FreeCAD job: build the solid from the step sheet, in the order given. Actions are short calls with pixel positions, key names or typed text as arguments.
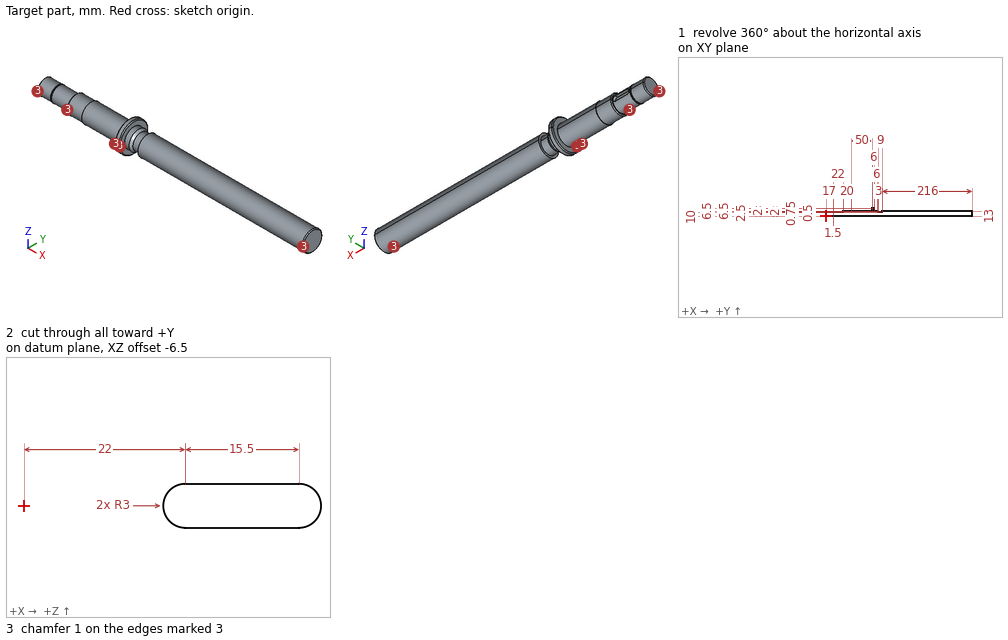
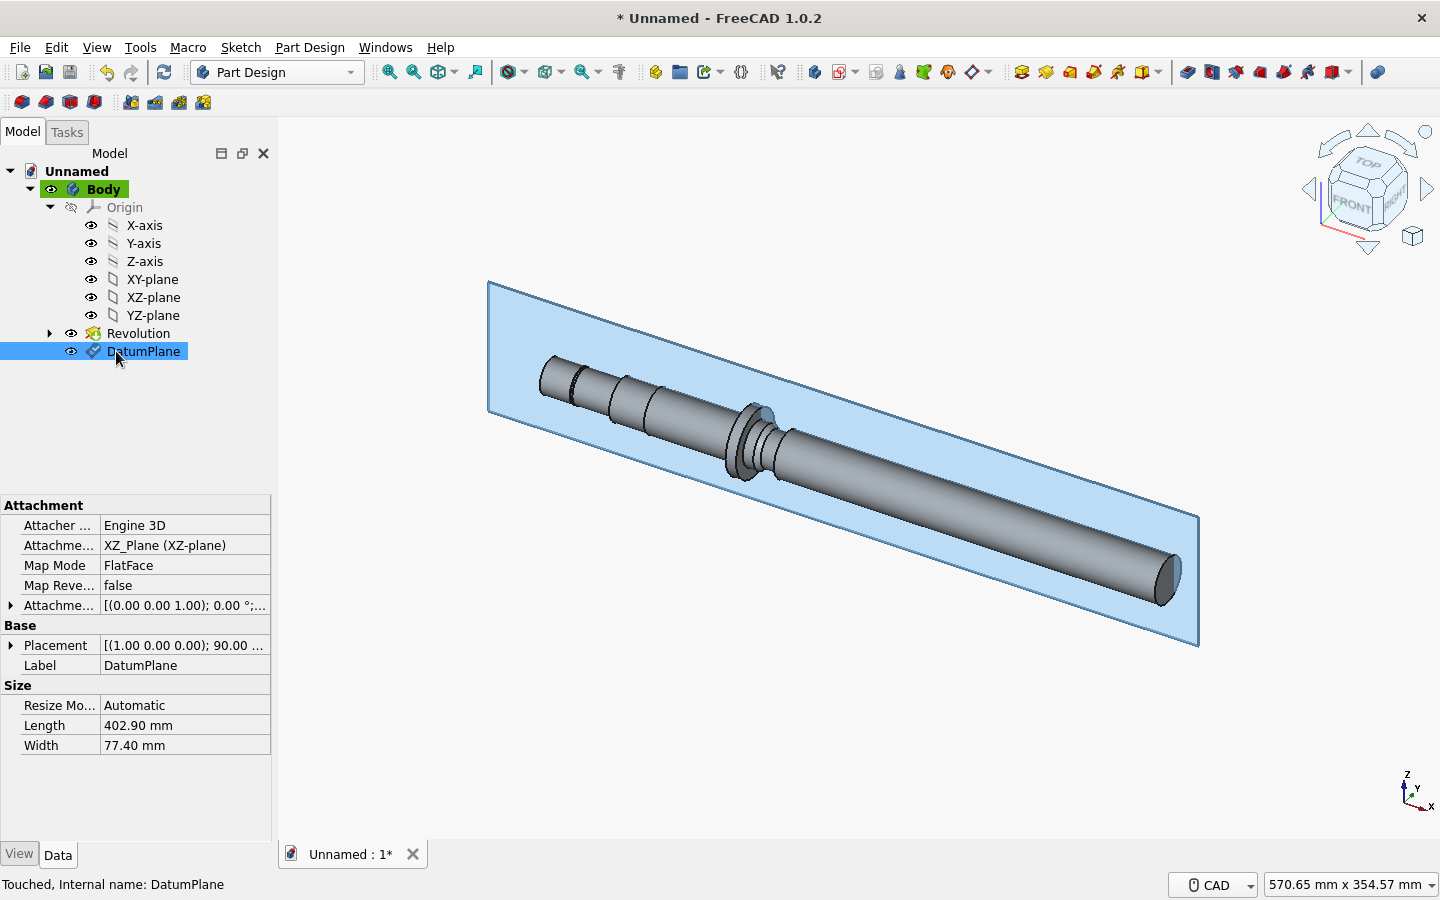
click(840, 72)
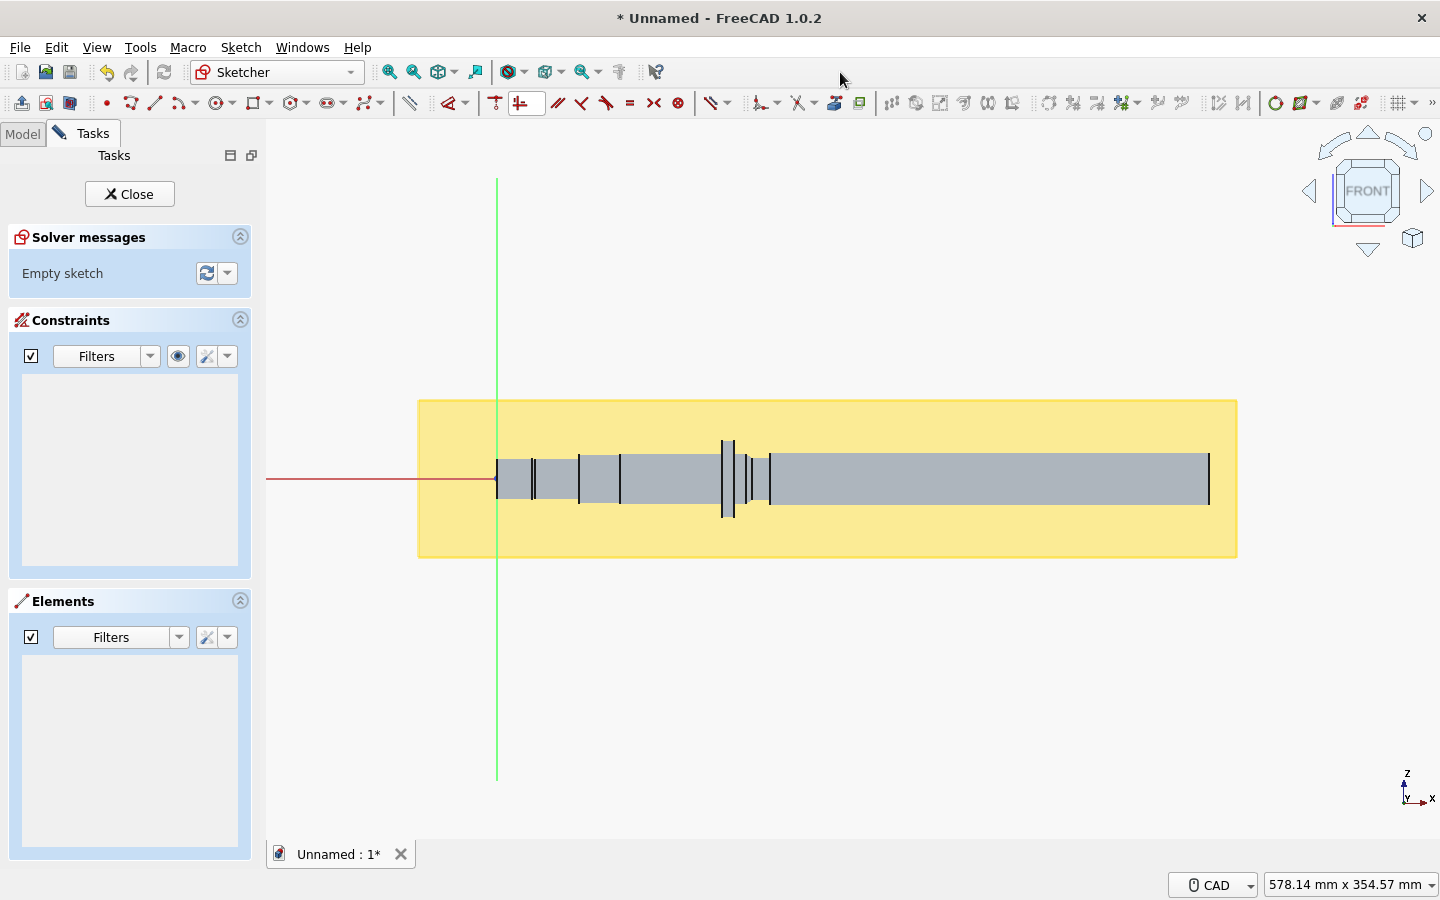
click(70, 104)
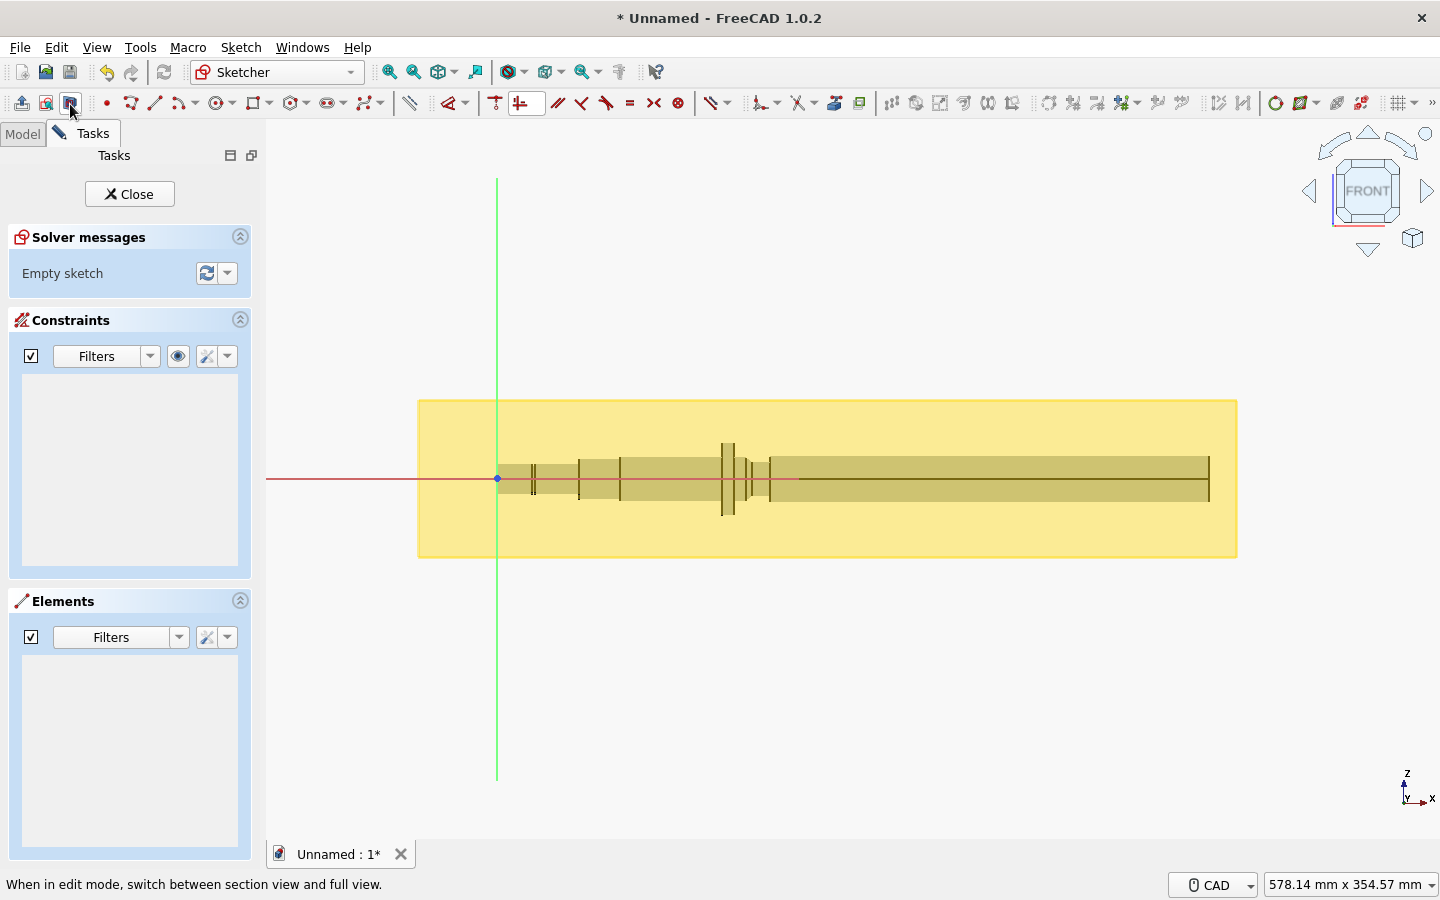
scroll(508, 479, up, 11)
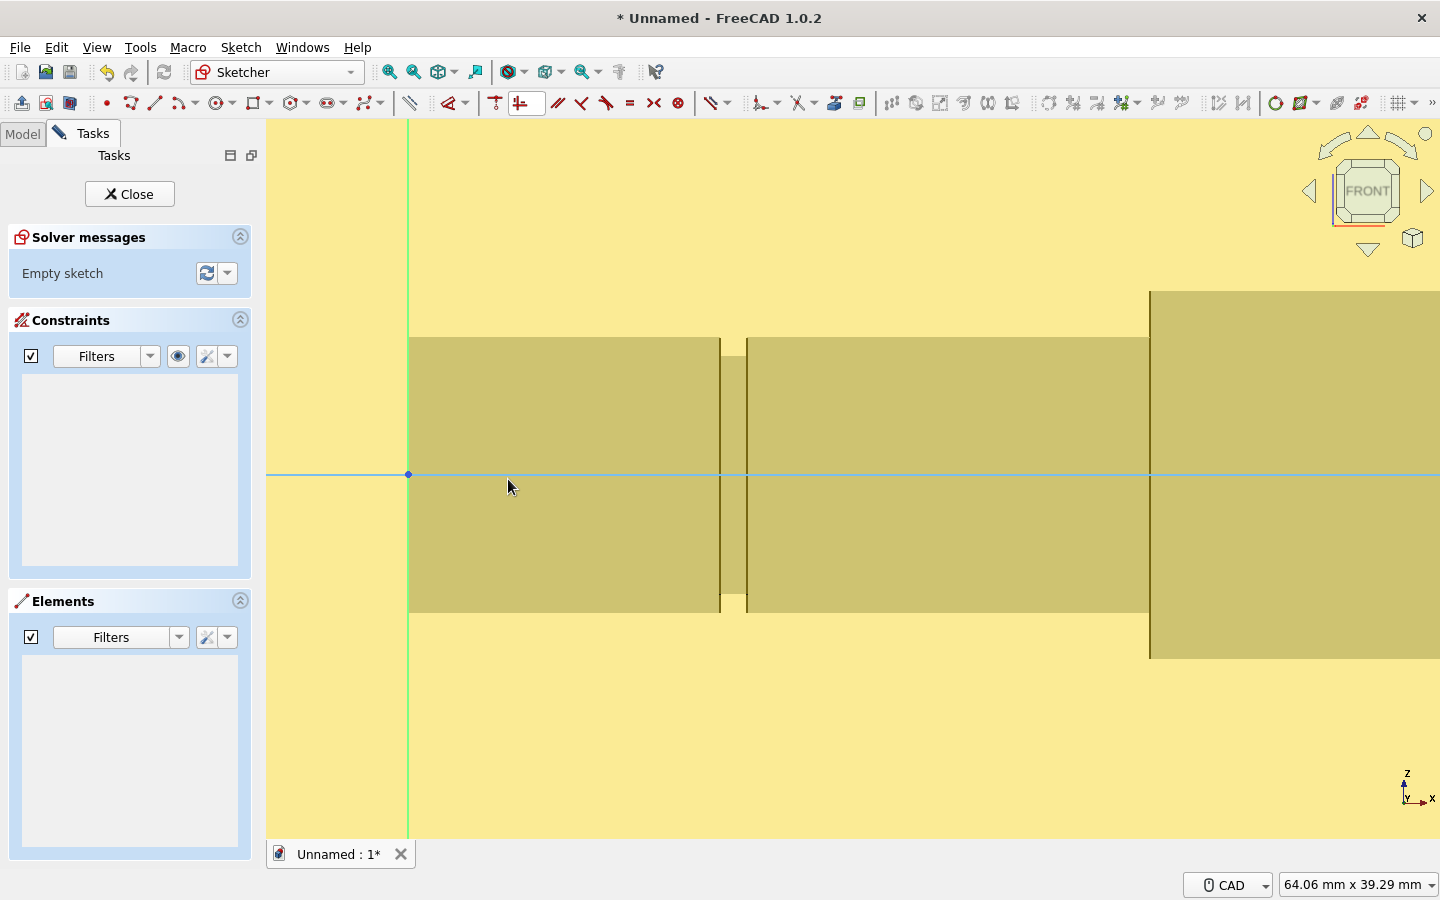
click(328, 104)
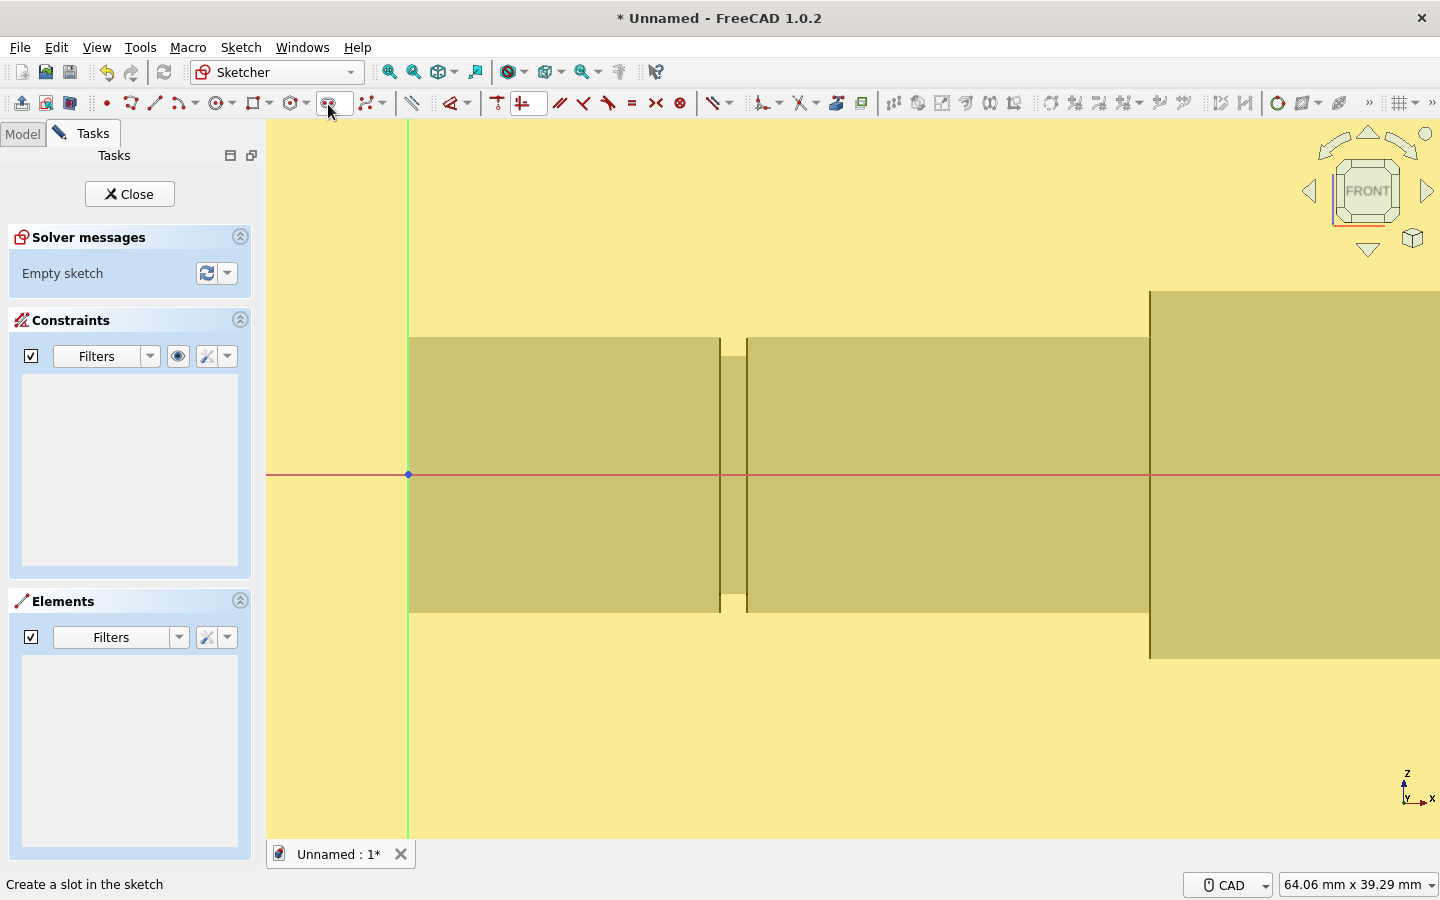
click(811, 475)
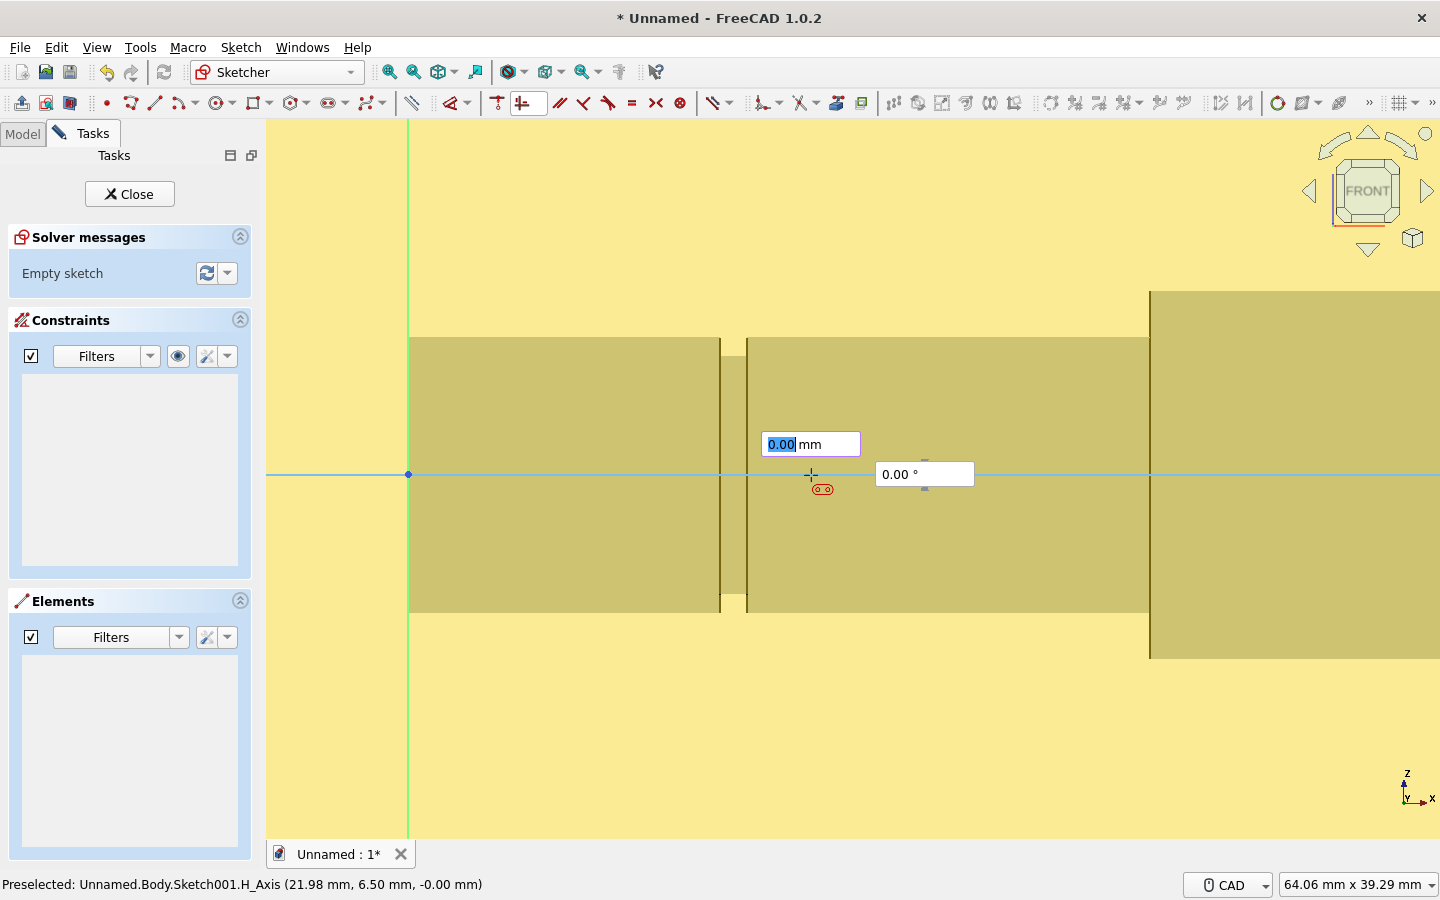
click(1095, 466)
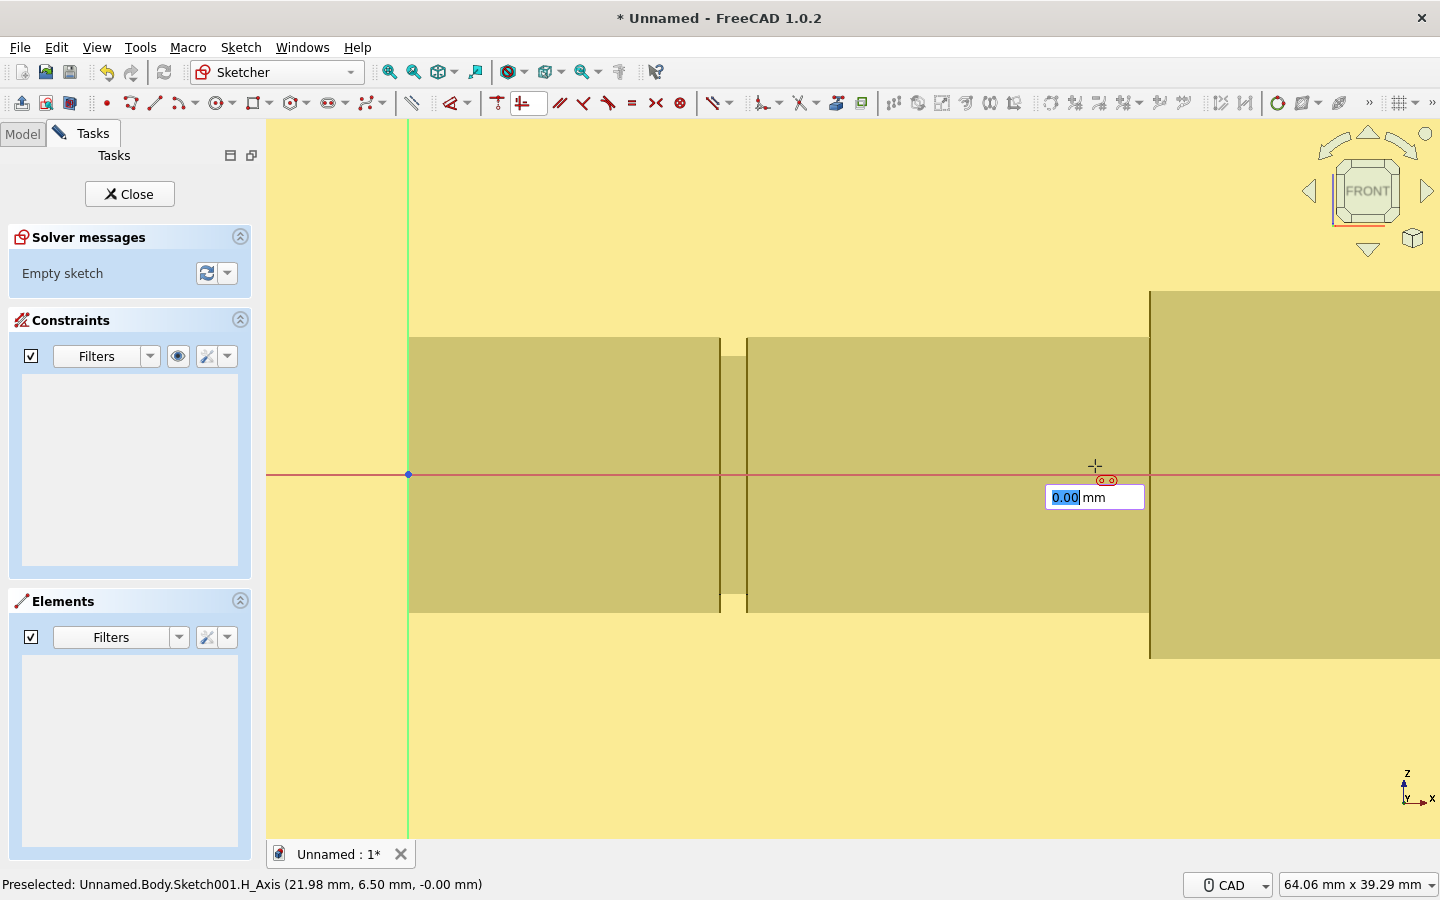
click(953, 530)
key(Escape)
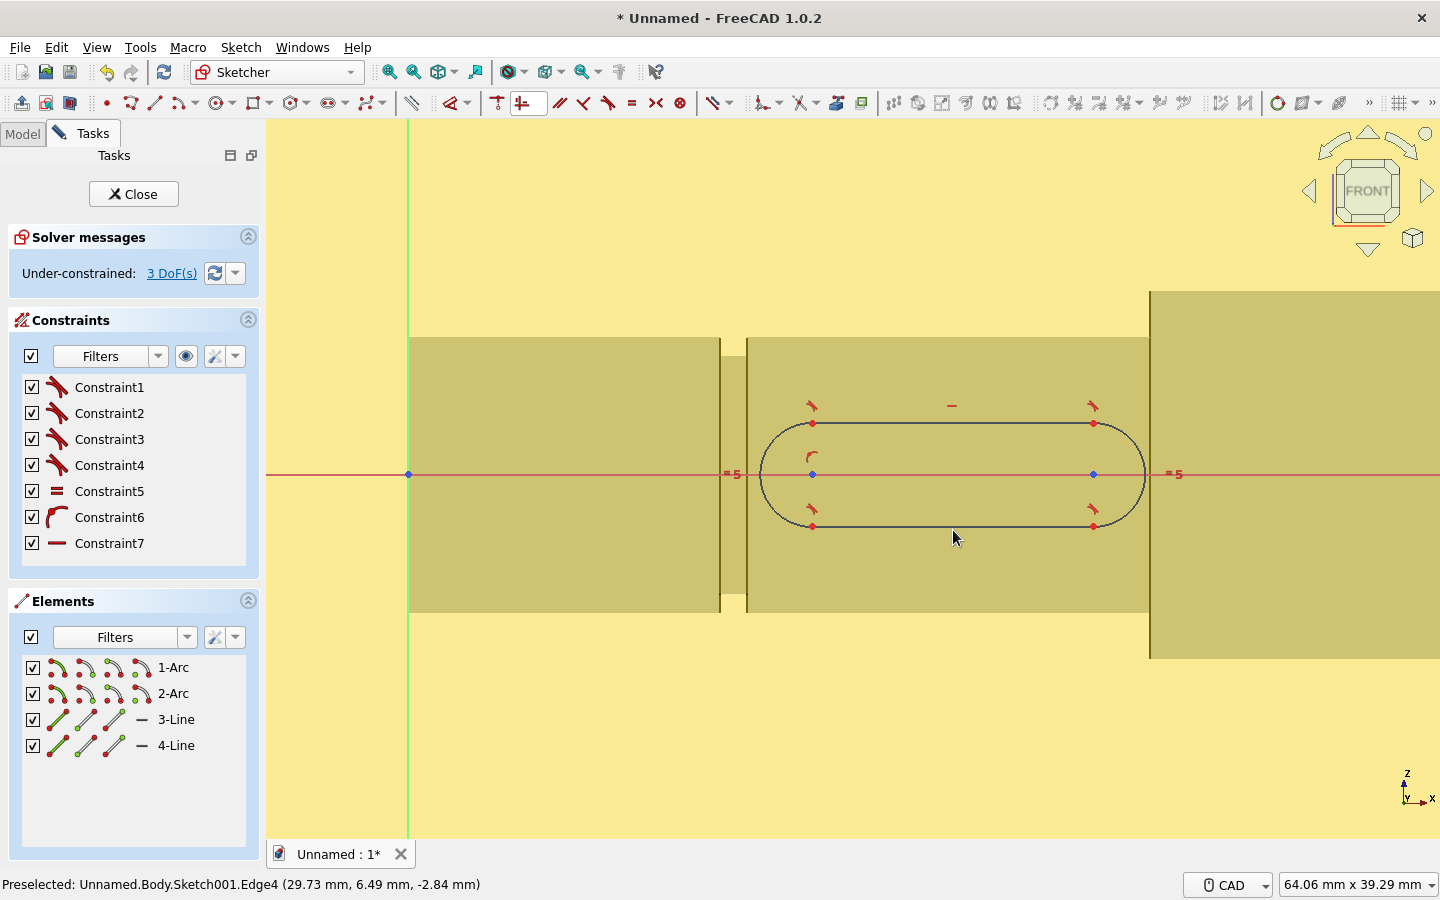
key(d)